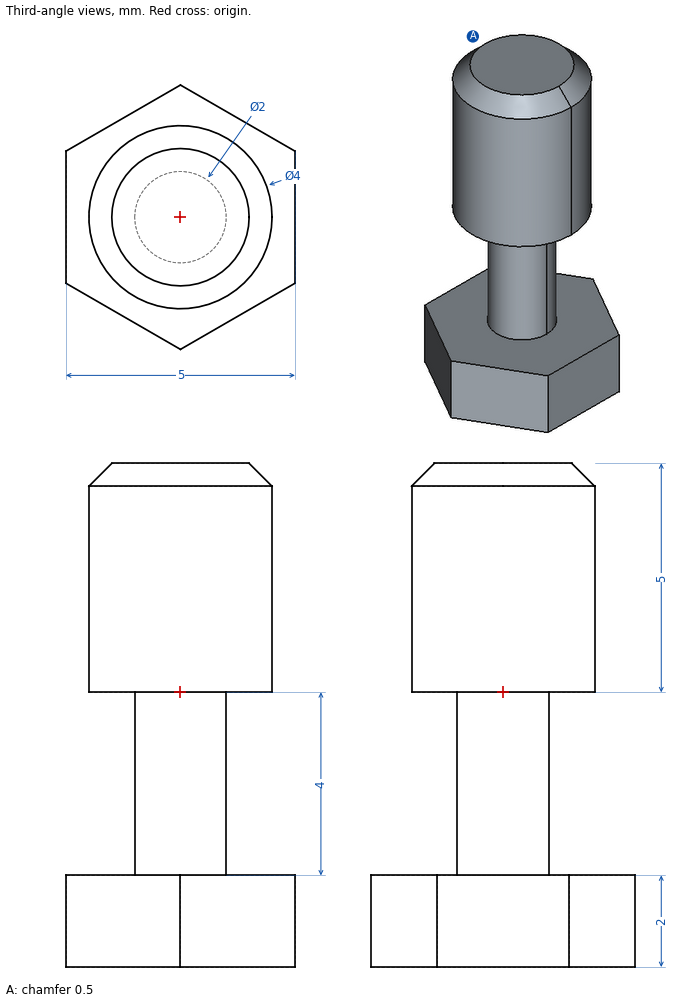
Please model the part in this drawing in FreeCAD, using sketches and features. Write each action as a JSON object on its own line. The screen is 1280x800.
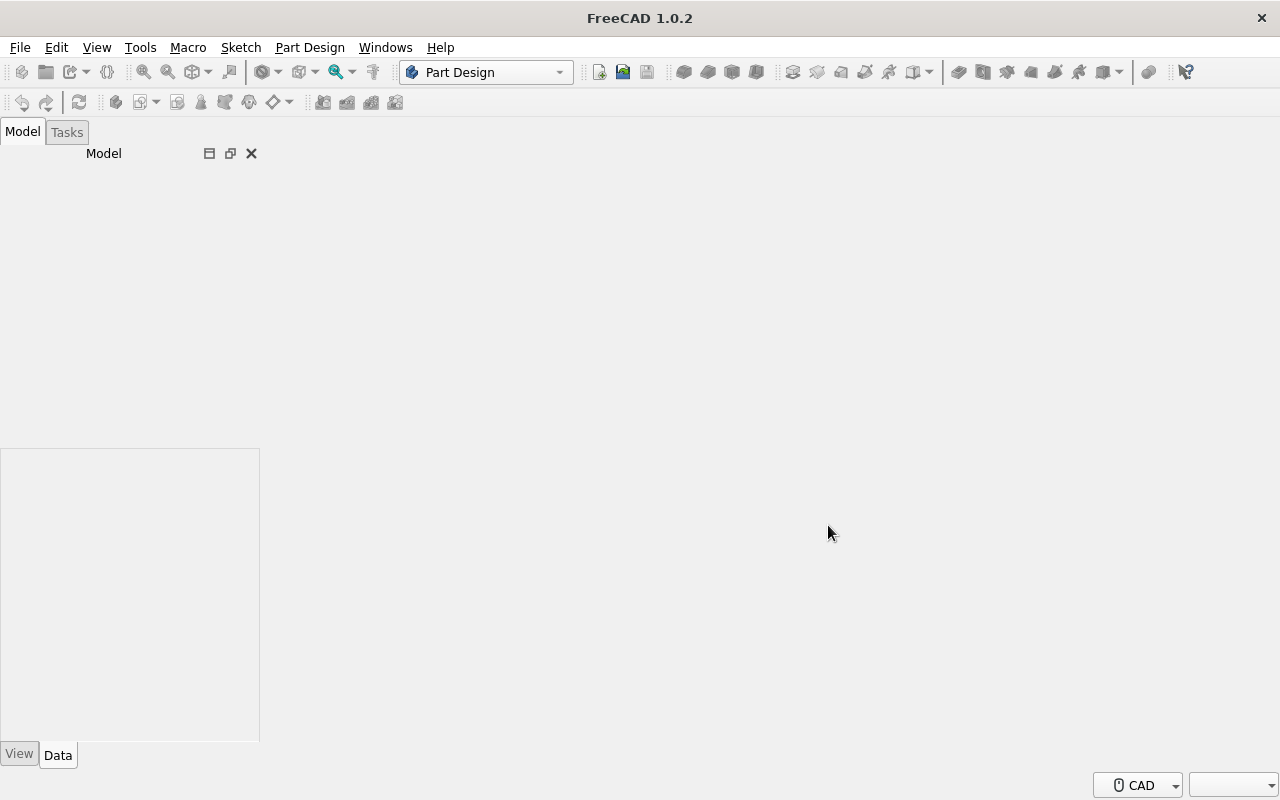
{"action": "left_click", "coordinate": [600, 72]}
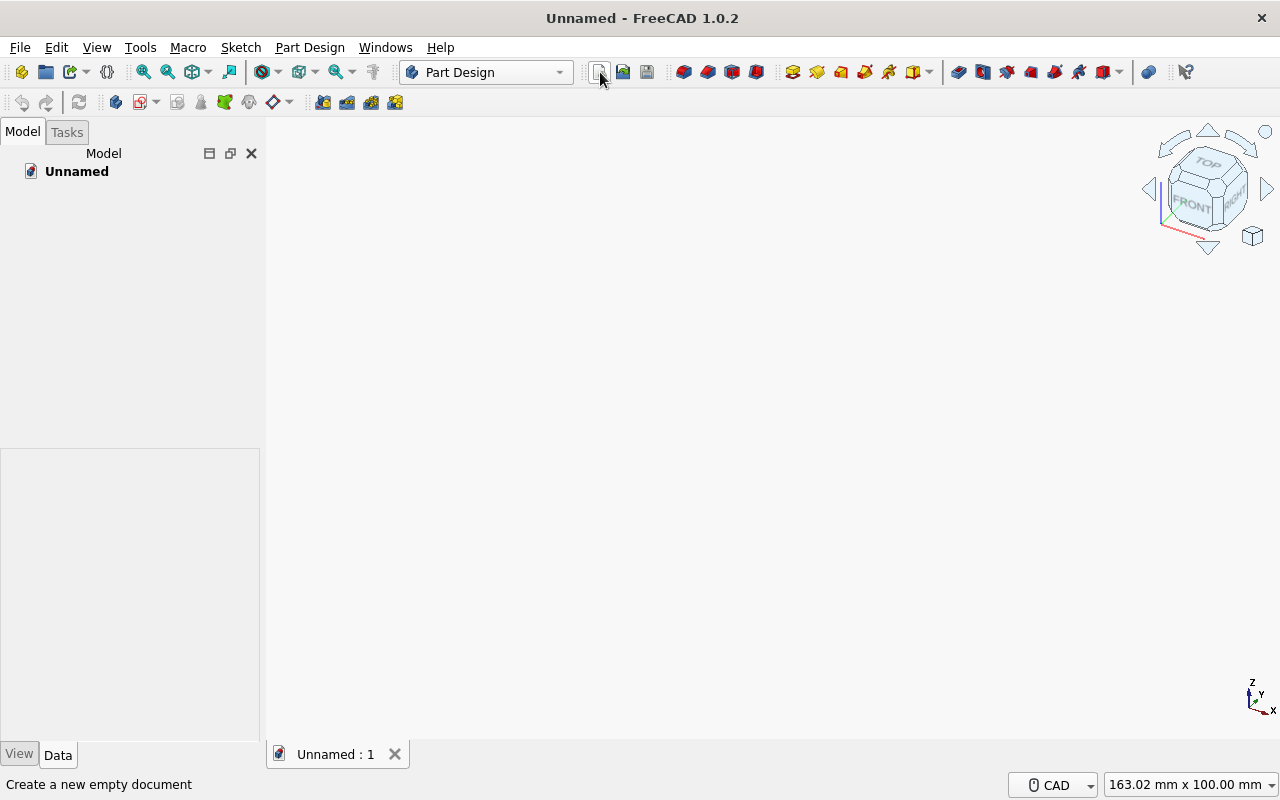
{"action": "left_click", "coordinate": [140, 102]}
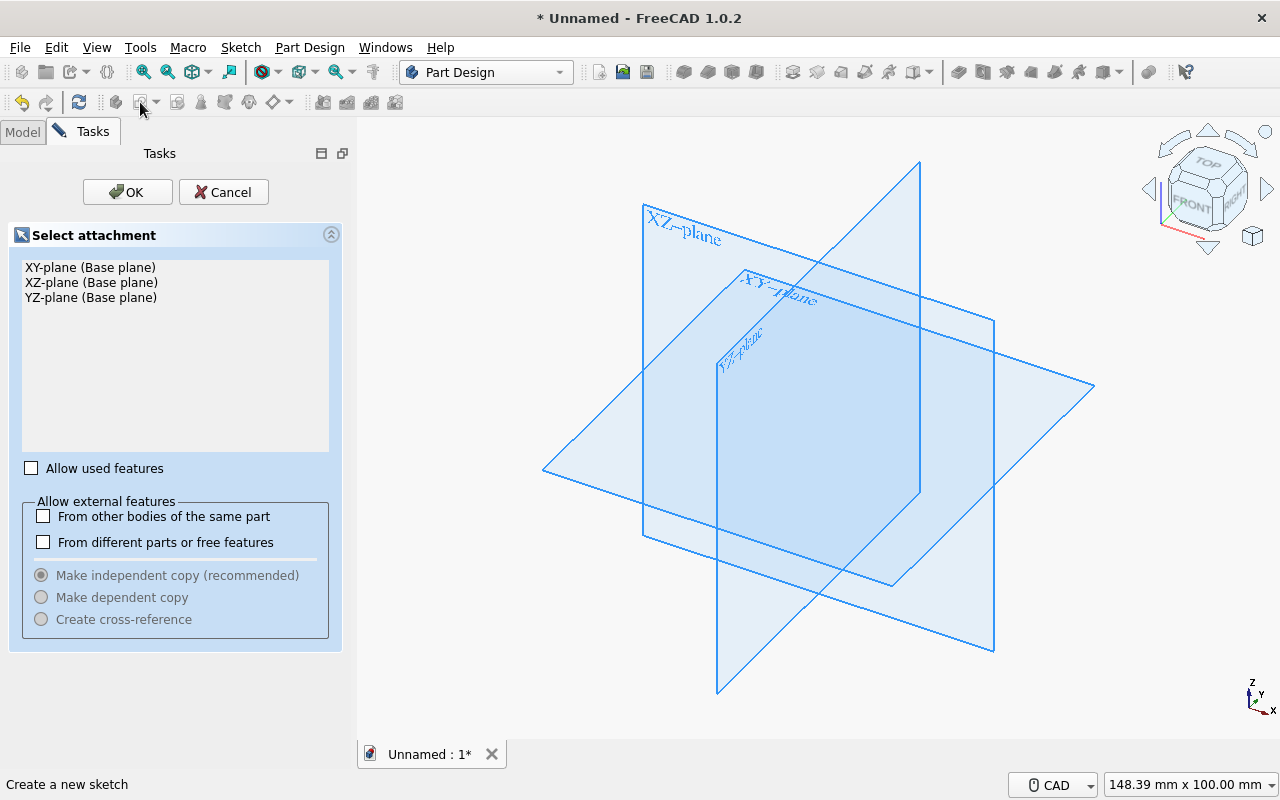
{"action": "left_click", "coordinate": [82, 268]}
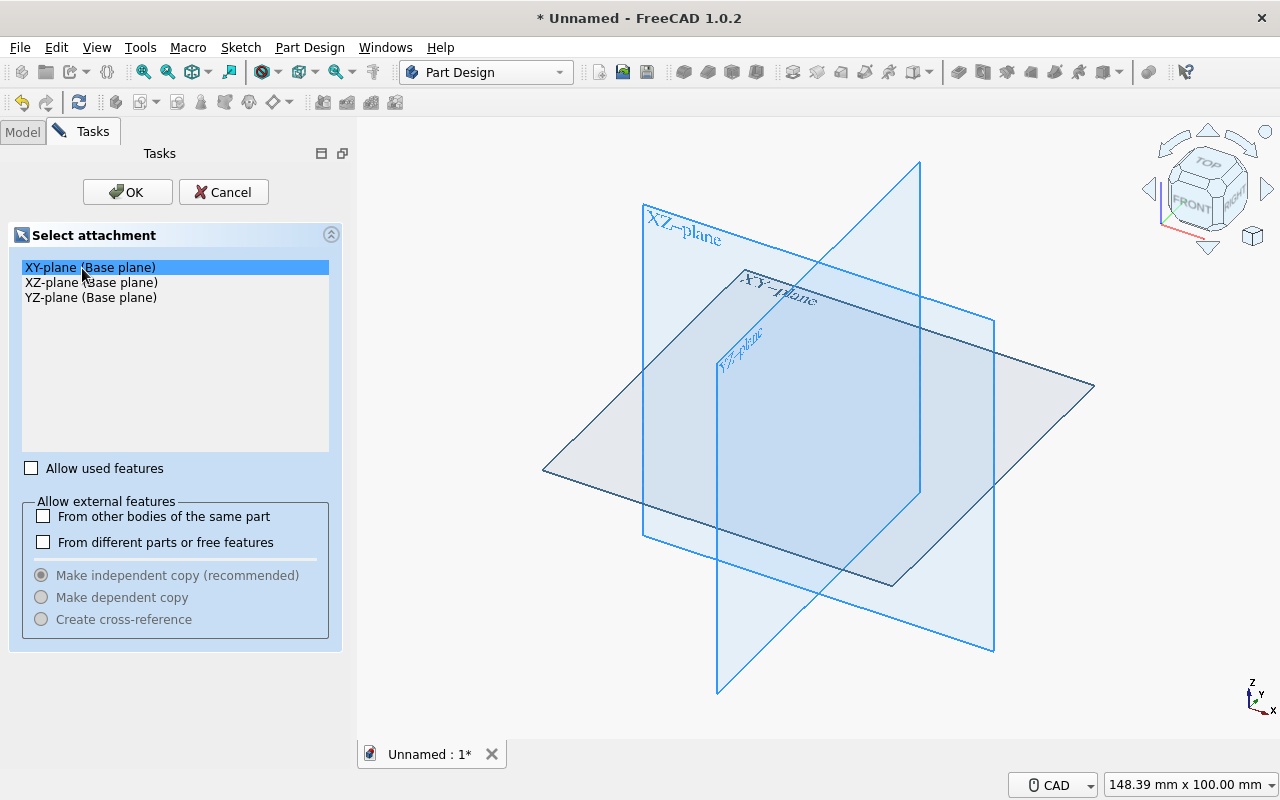
{"action": "left_click", "coordinate": [128, 192]}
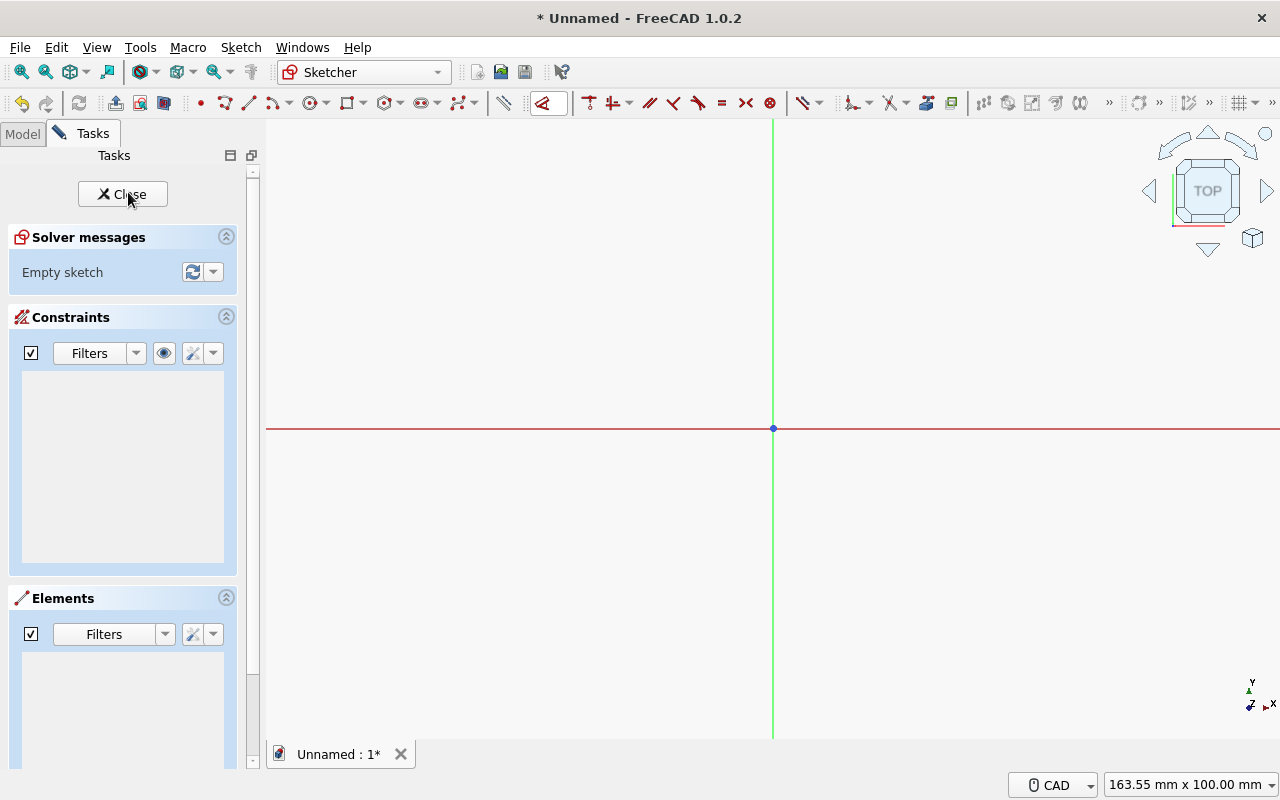
{"action": "scroll", "coordinate": [777, 429], "scroll_direction": "up", "scroll_amount": 14}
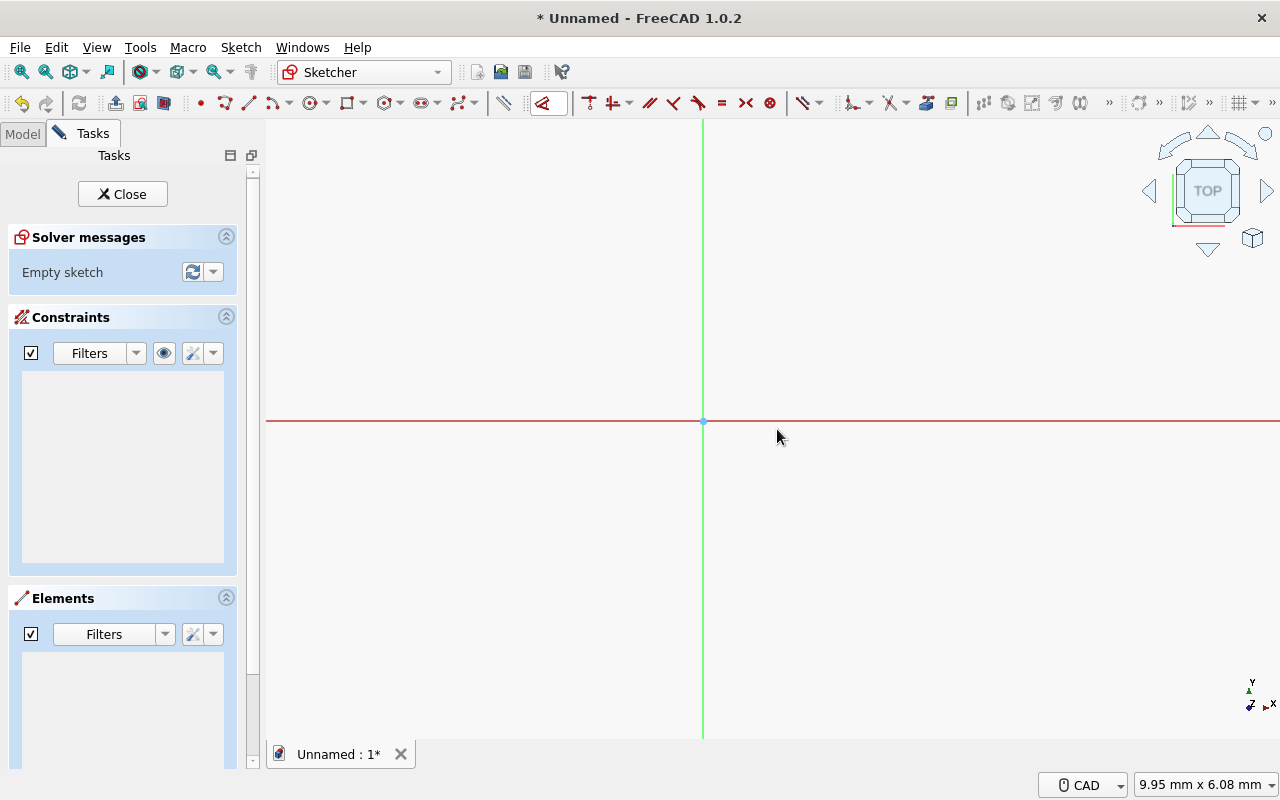
{"action": "left_click", "coordinate": [310, 104]}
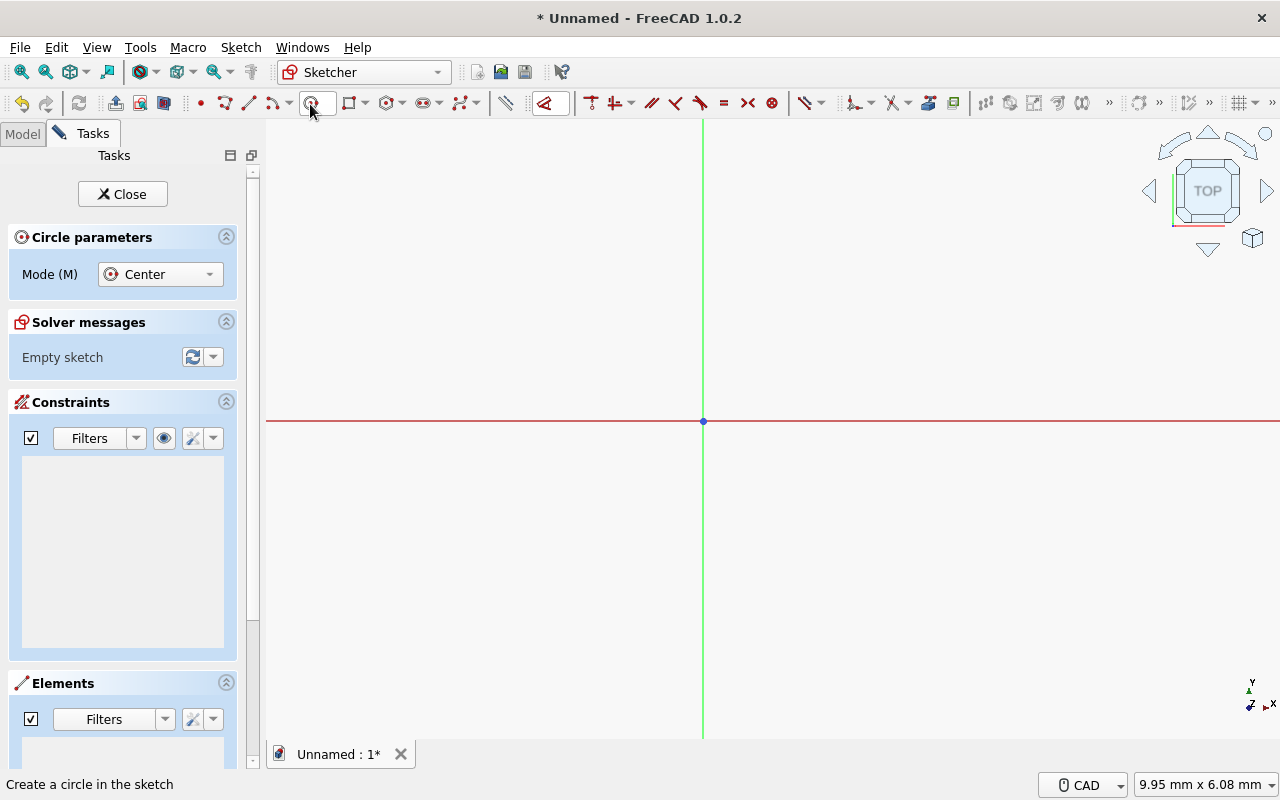
{"action": "left_click", "coordinate": [703, 421]}
{"action": "left_click", "coordinate": [848, 277]}
{"action": "key", "text": "Escape"}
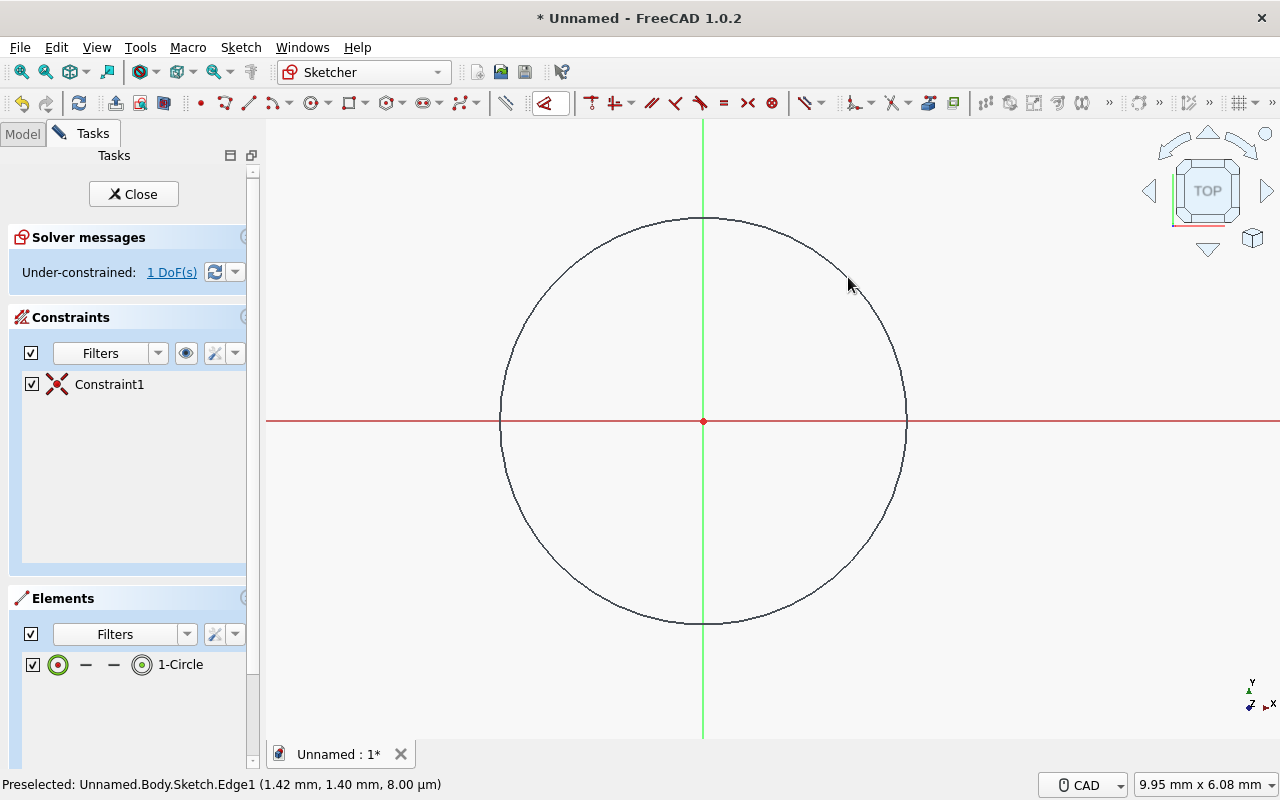
{"action": "left_click", "coordinate": [544, 104]}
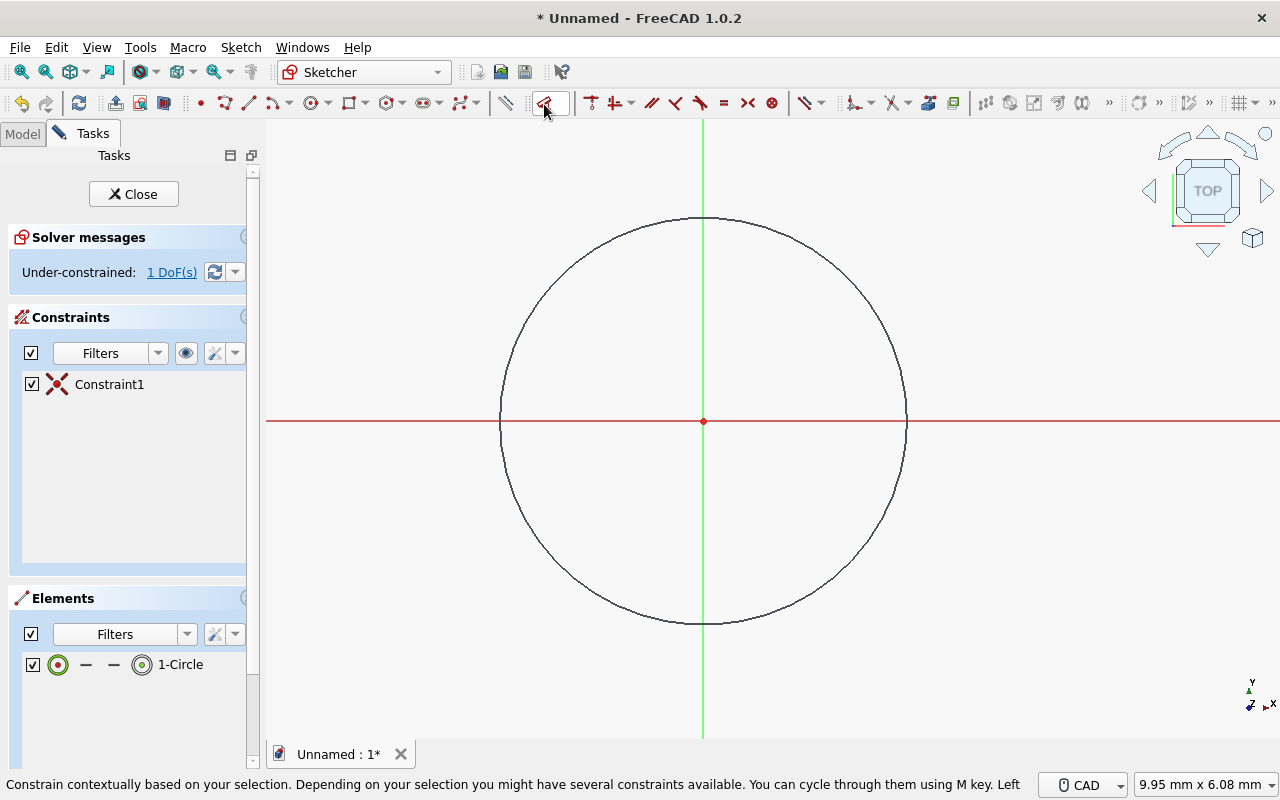
{"action": "left_click", "coordinate": [847, 277]}
{"action": "left_click", "coordinate": [870, 254]}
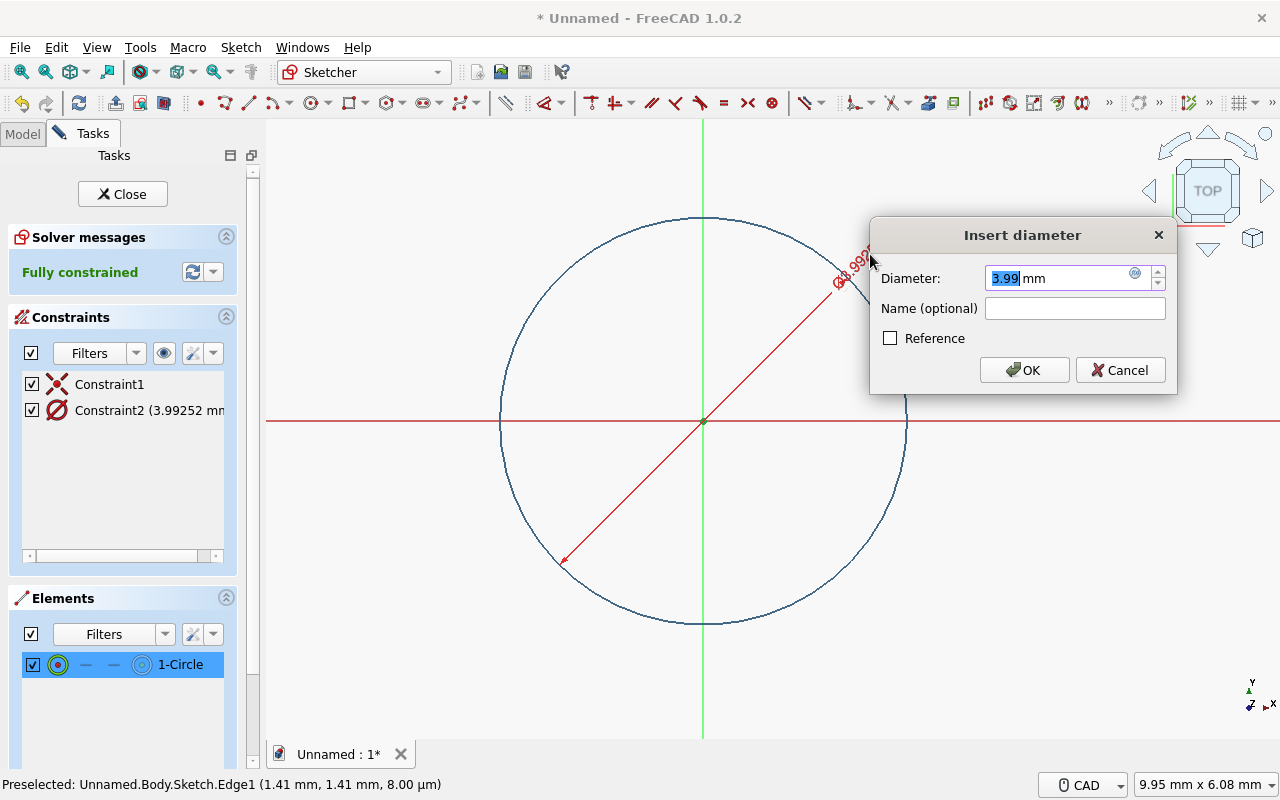
{"action": "type", "text": "4"}
{"action": "key", "text": "Return"}
{"action": "key", "text": "Escape"}